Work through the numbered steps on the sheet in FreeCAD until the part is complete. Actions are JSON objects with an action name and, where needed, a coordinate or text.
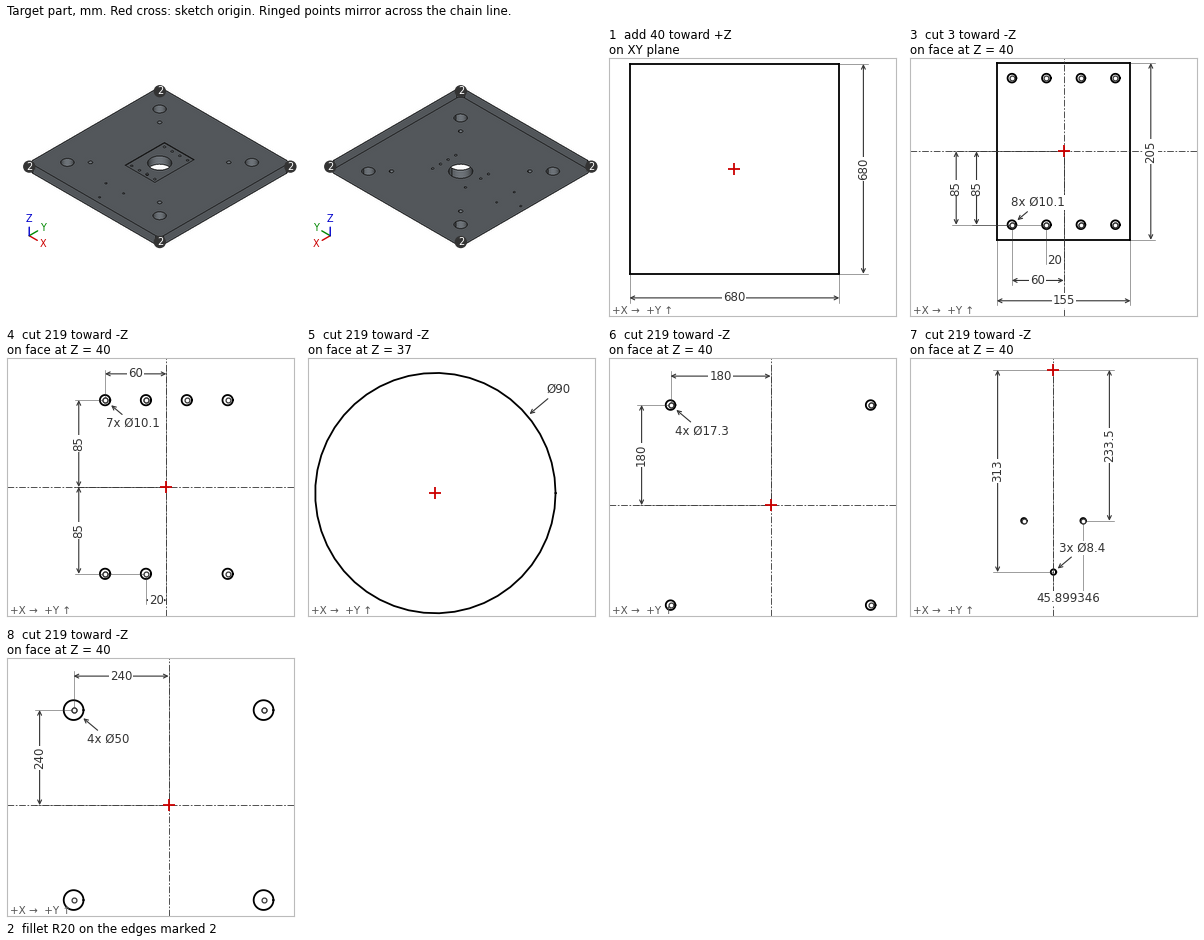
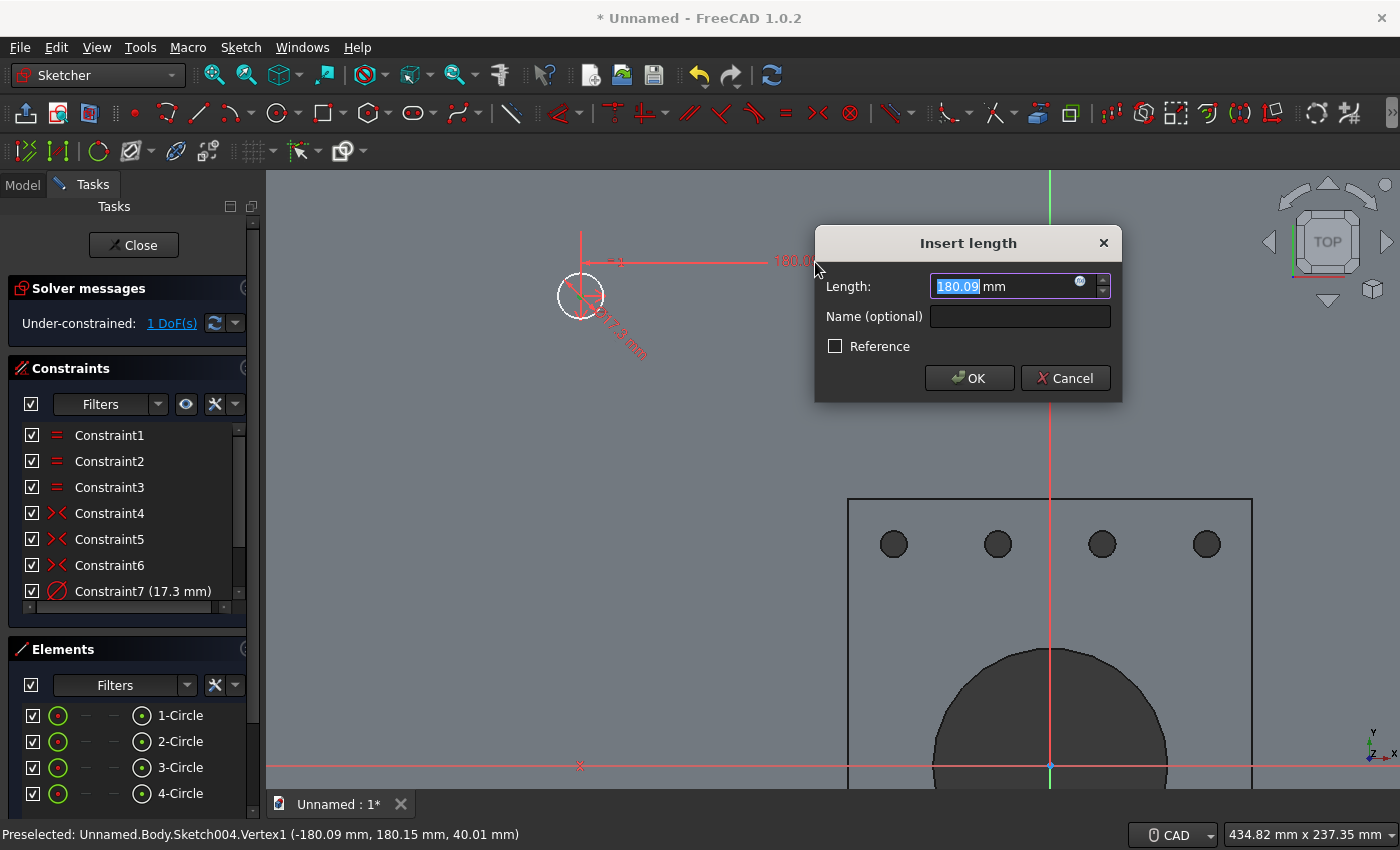
{"action": "type", "text": "180"}
{"action": "key", "text": "Return"}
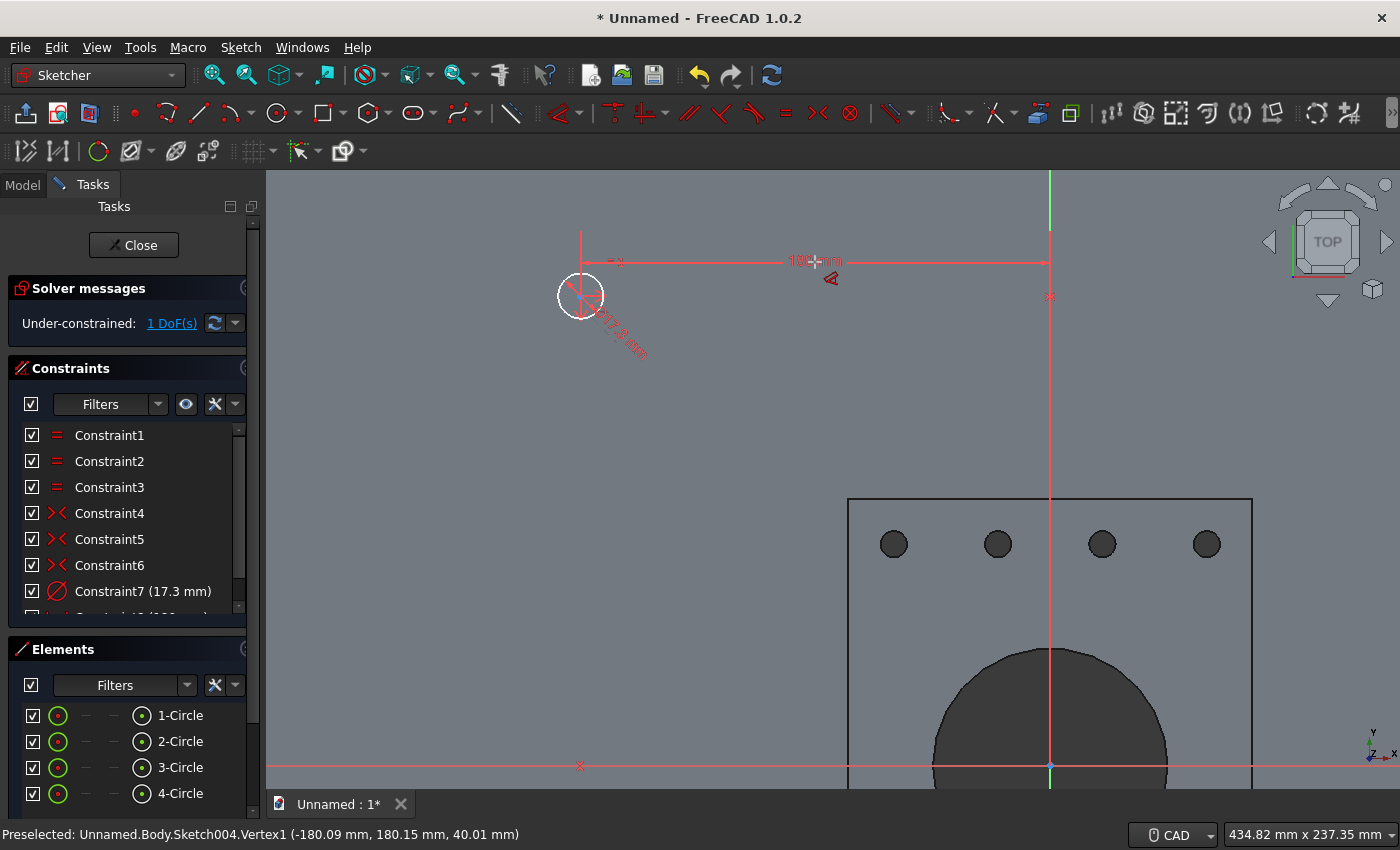
{"action": "left_click", "coordinate": [581, 296]}
{"action": "left_click", "coordinate": [547, 529]}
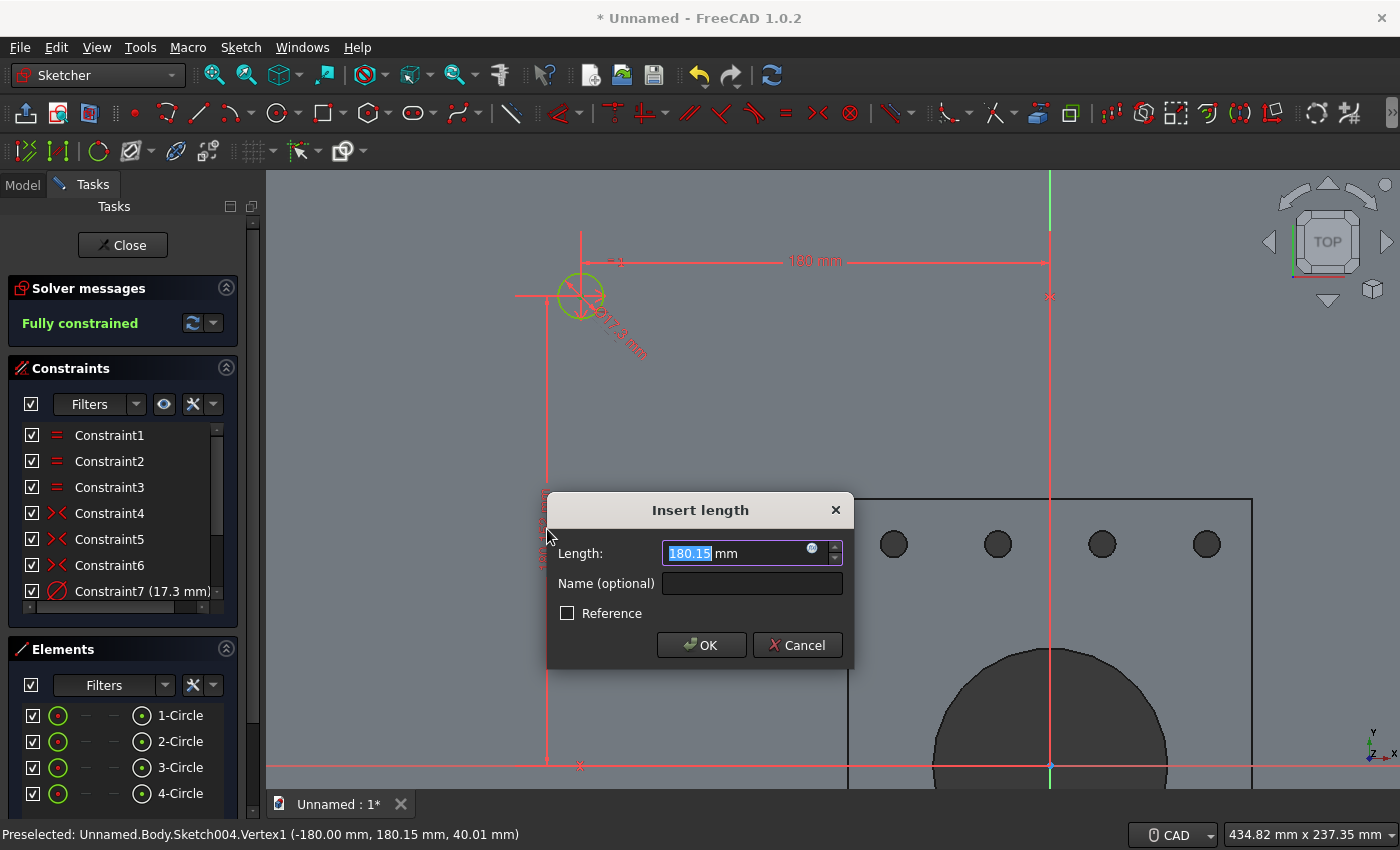
{"action": "type", "text": "180"}
{"action": "key", "text": "Return"}
{"action": "key", "text": "Escape"}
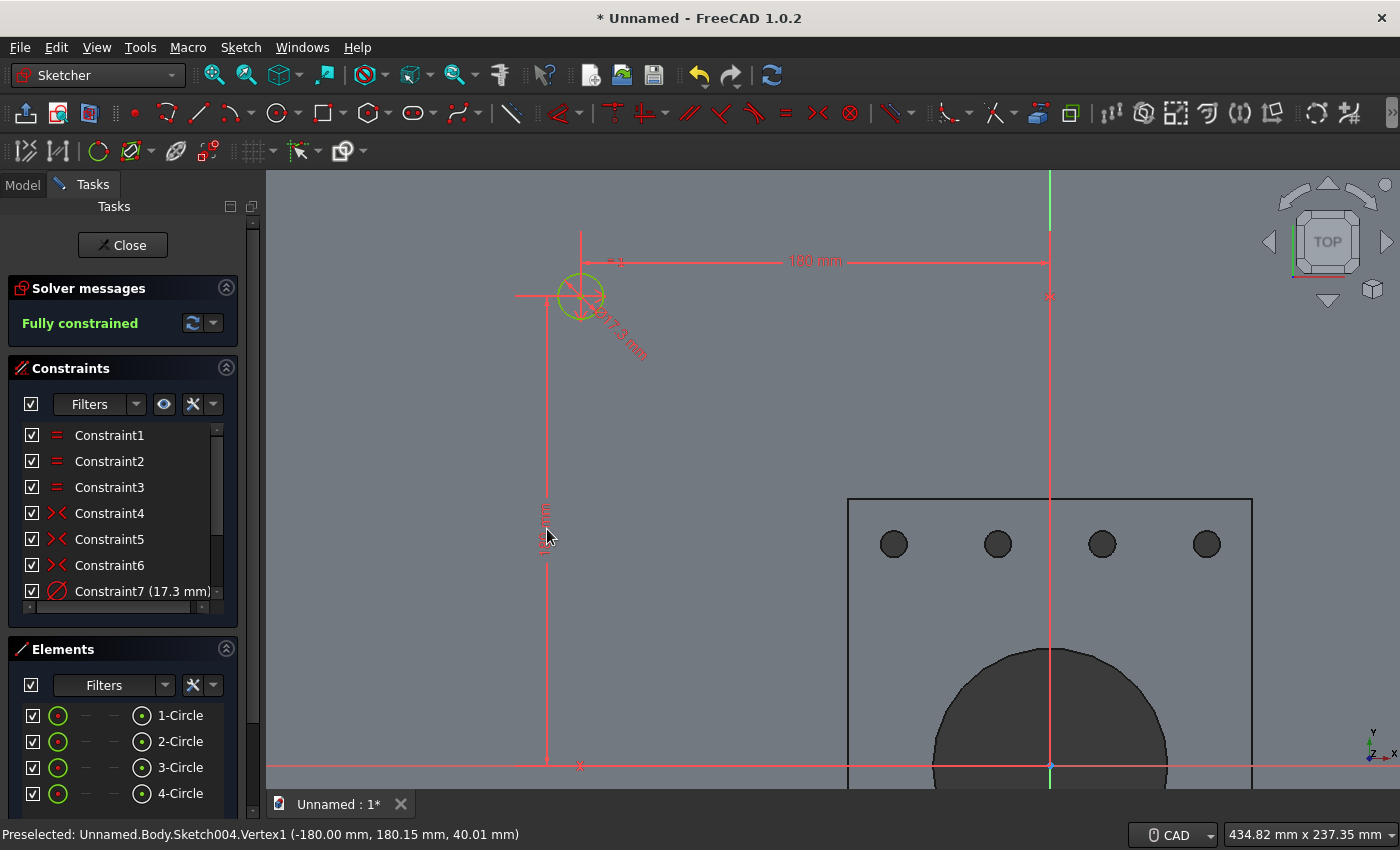
{"action": "left_click", "coordinate": [123, 245]}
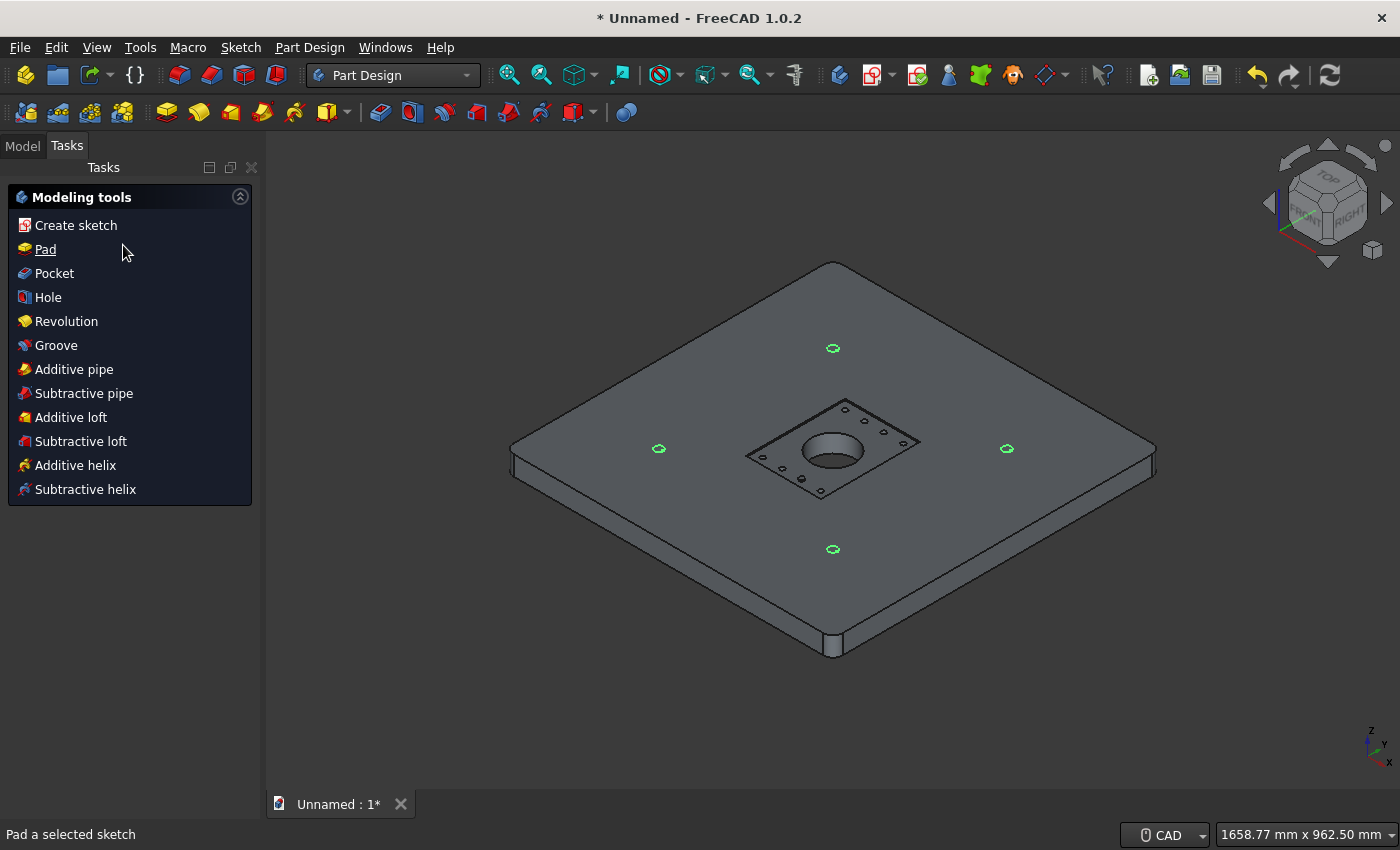
{"action": "left_click", "coordinate": [382, 112]}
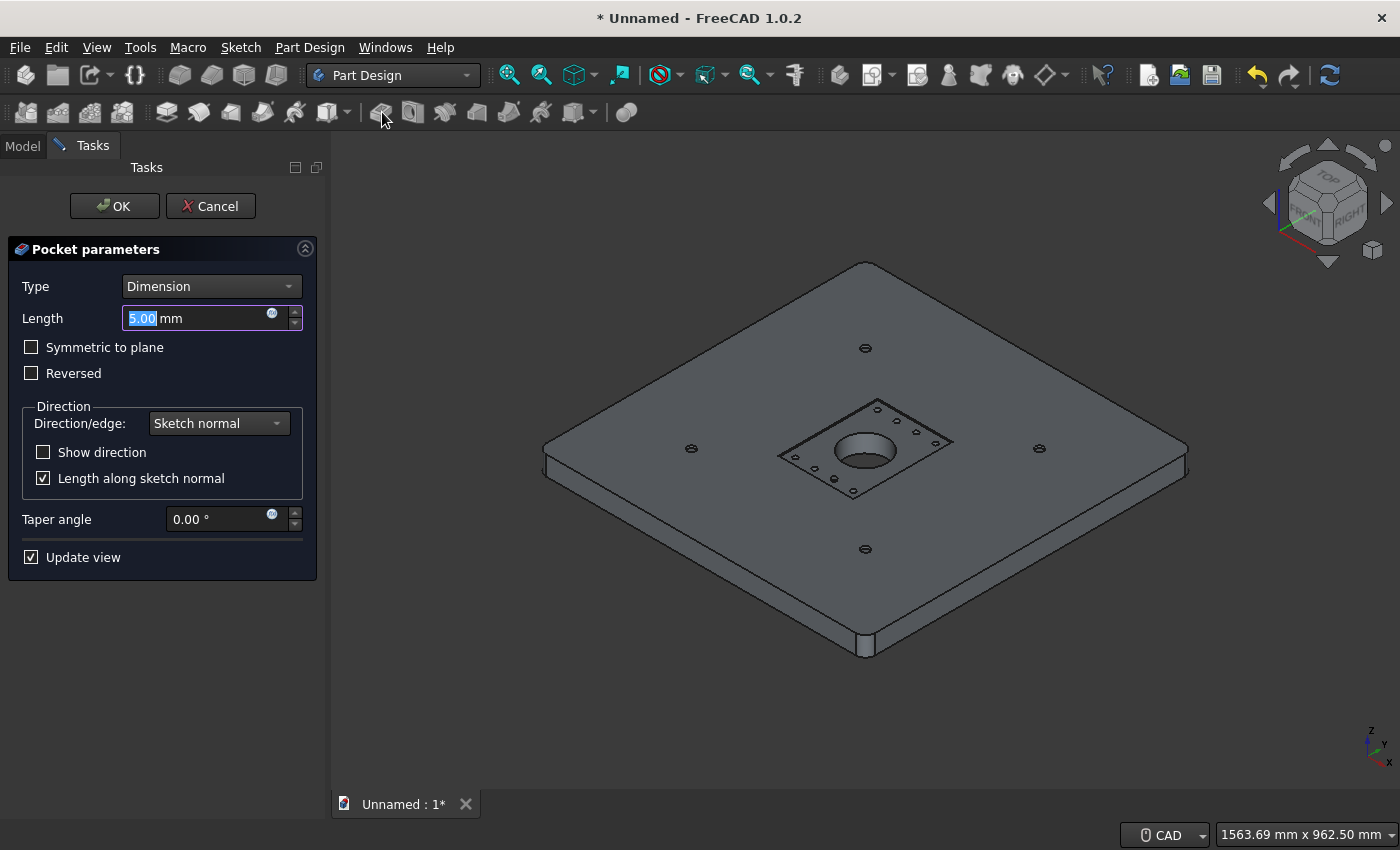
{"action": "type", "text": "219"}
{"action": "key", "text": "Tab"}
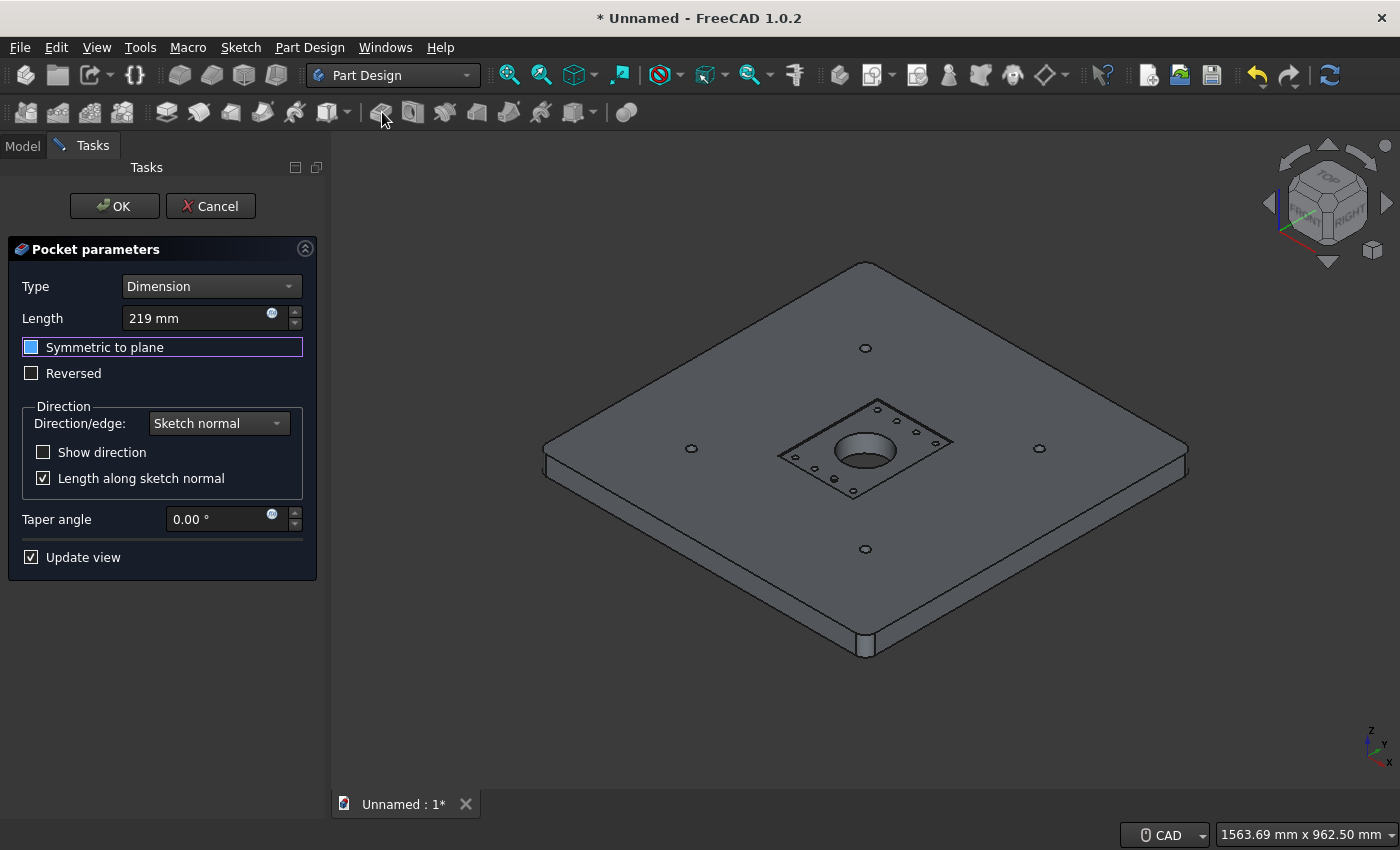
{"action": "left_click", "coordinate": [115, 206]}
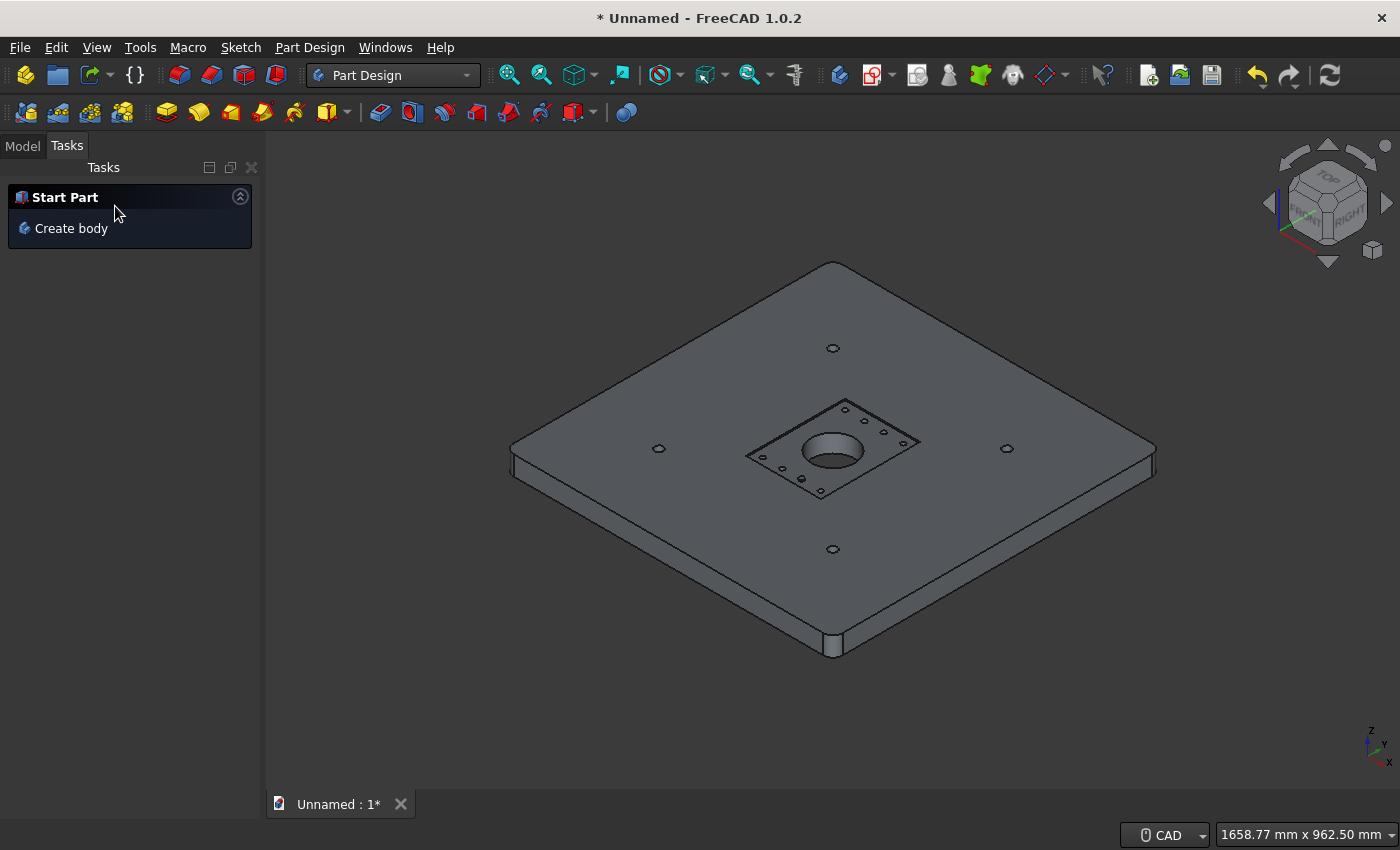
{"action": "left_click", "coordinate": [927, 502]}